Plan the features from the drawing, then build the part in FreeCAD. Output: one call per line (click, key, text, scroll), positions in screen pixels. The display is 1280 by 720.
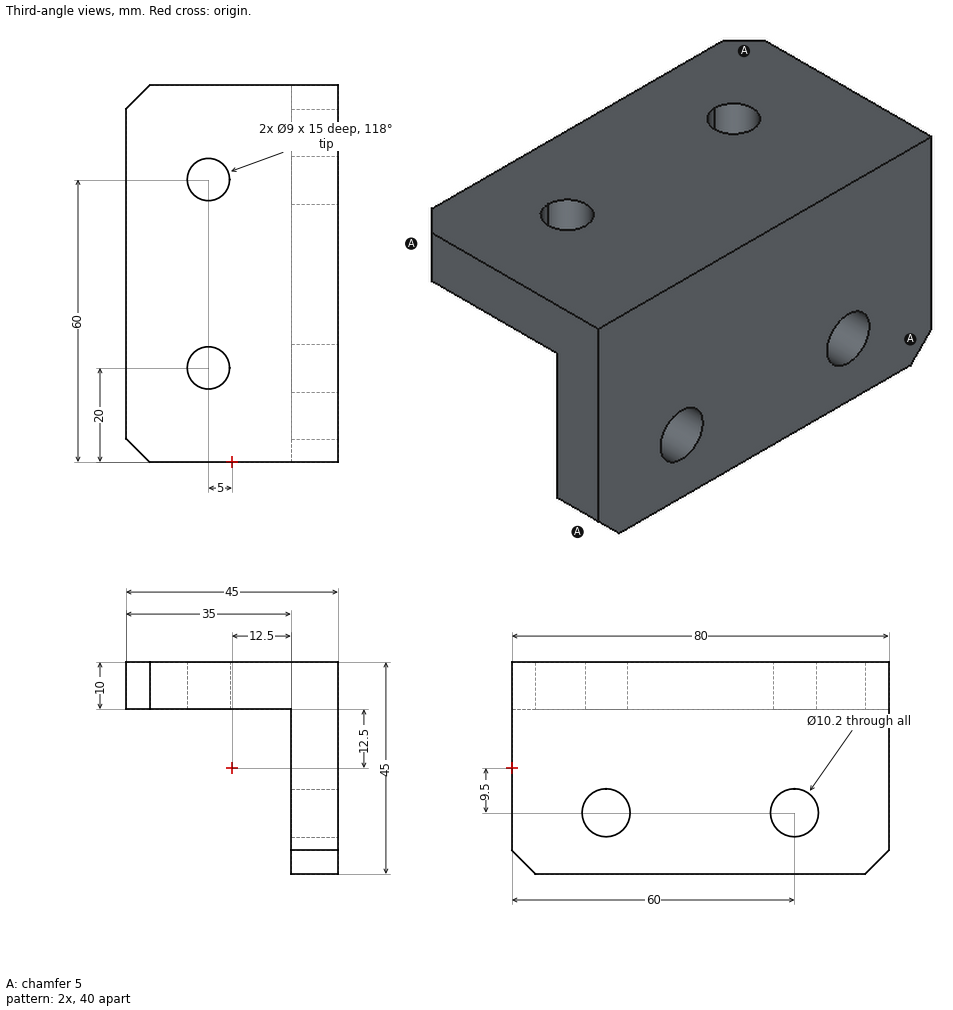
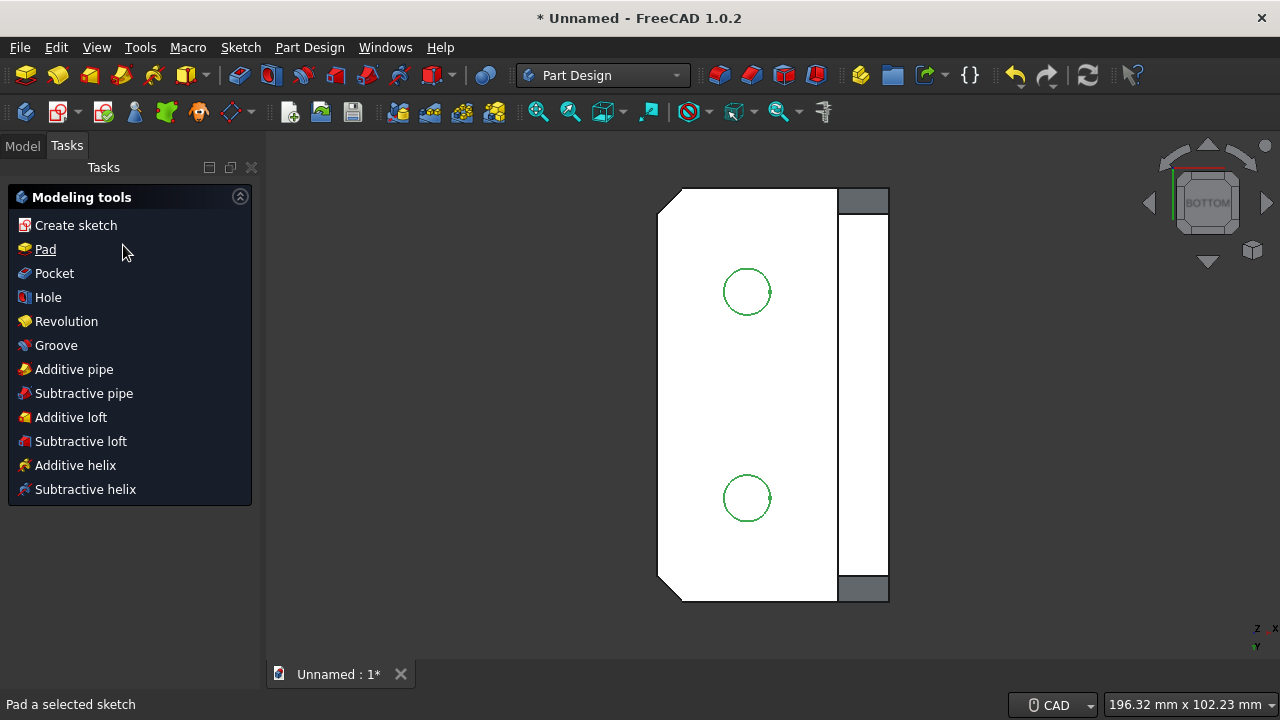
click(272, 76)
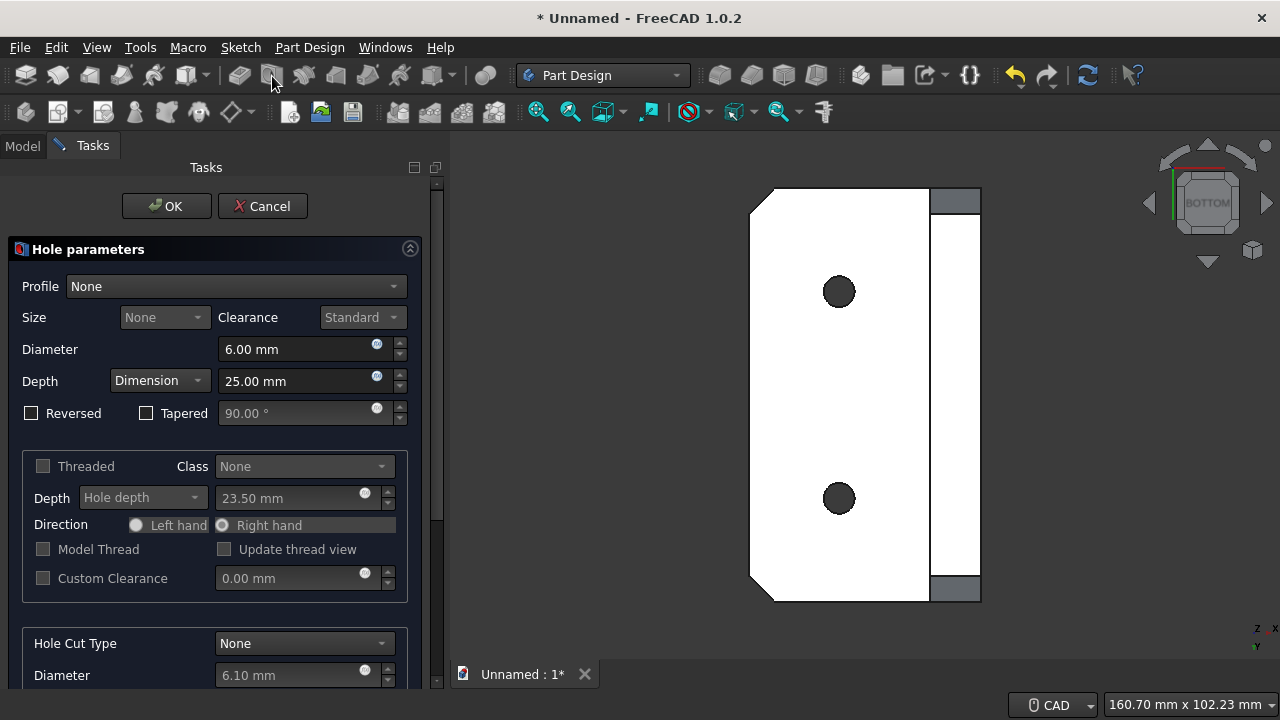
triple_click(305, 349)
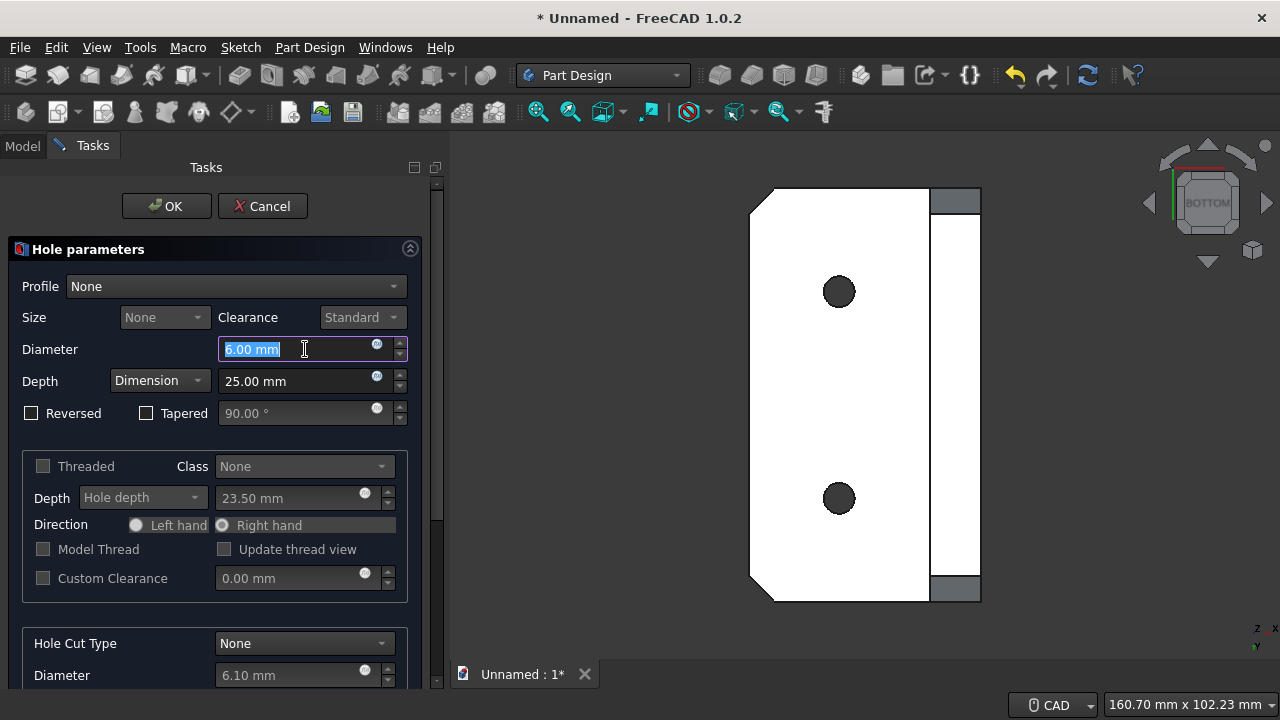
text(9)
key(Tab)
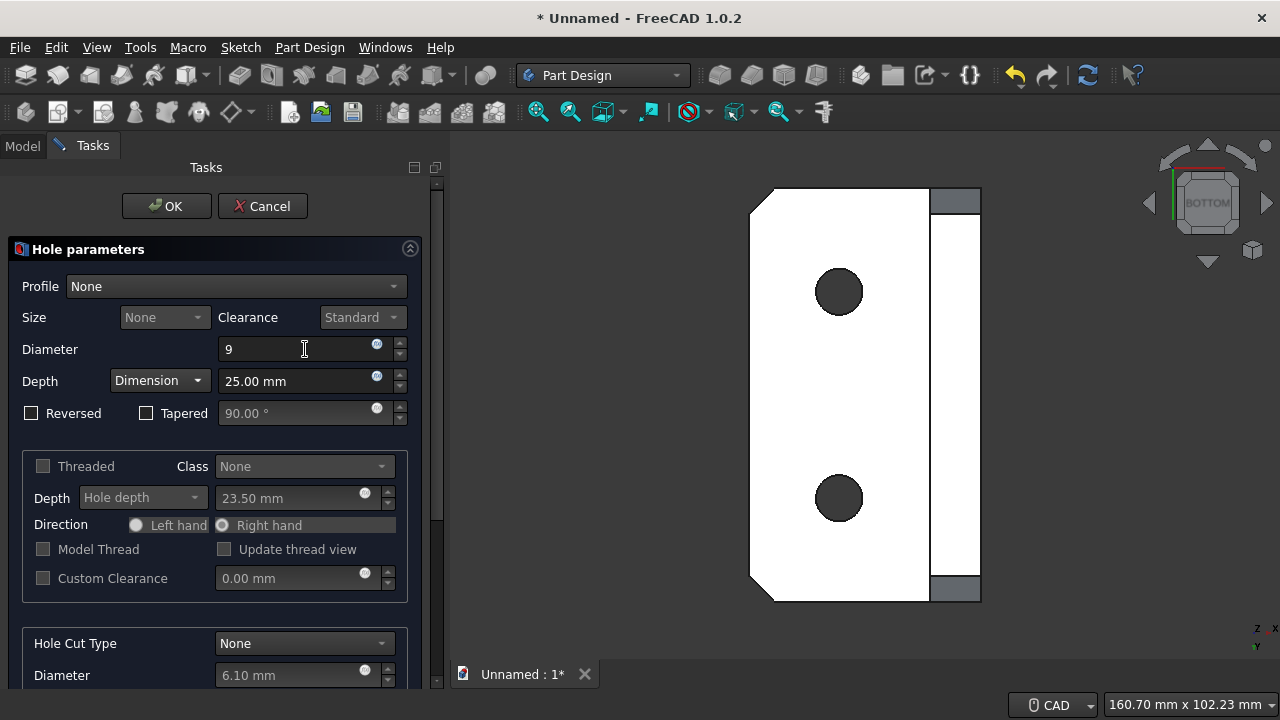
triple_click(305, 381)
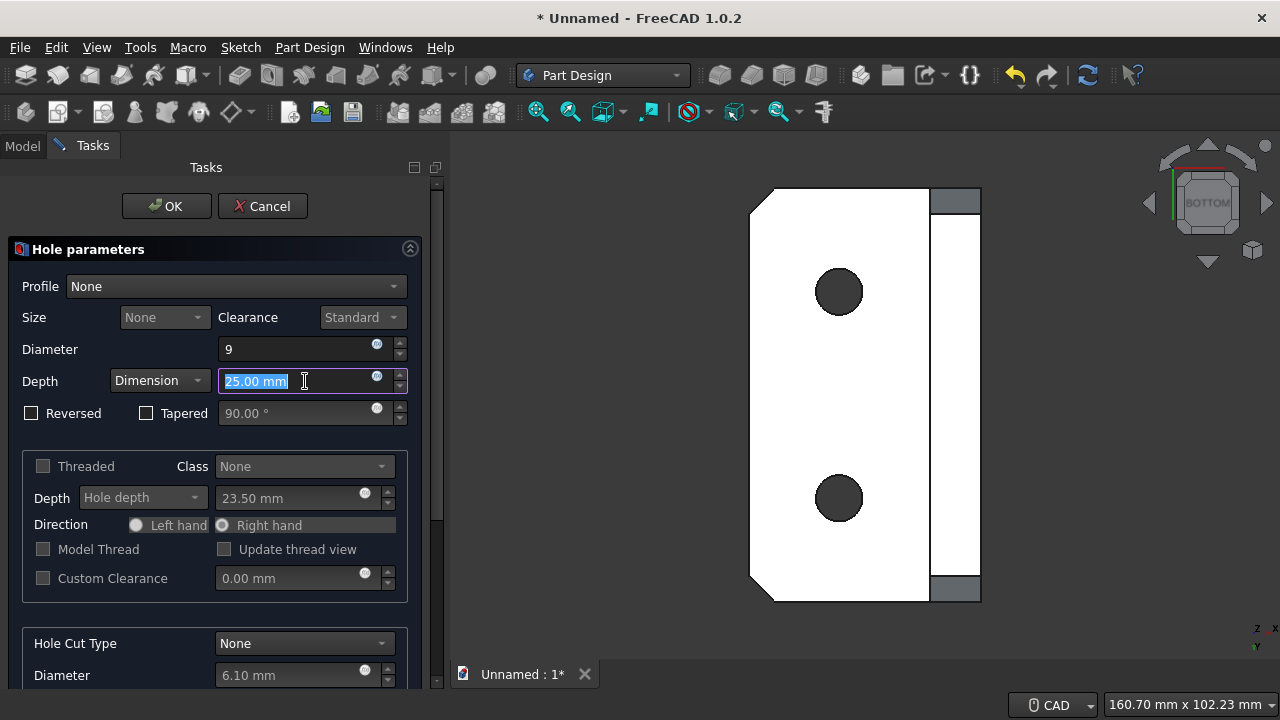
text(15)
key(Tab)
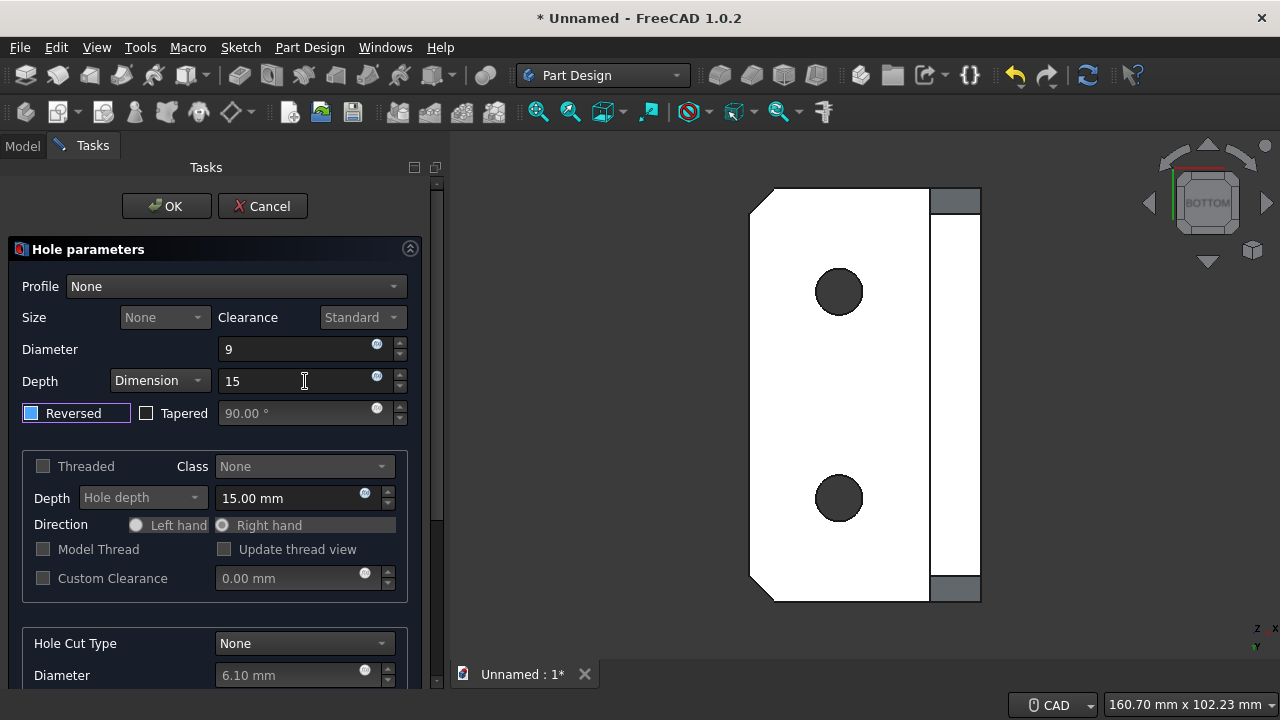
click(167, 206)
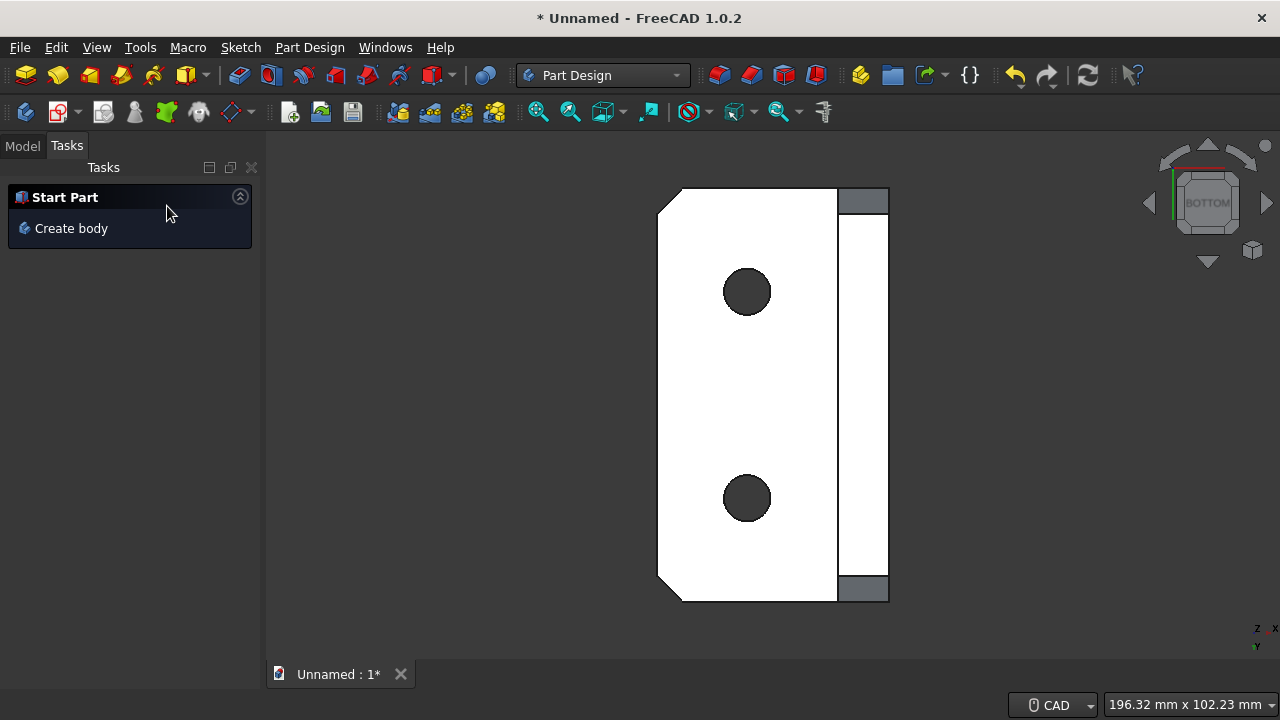
key(6)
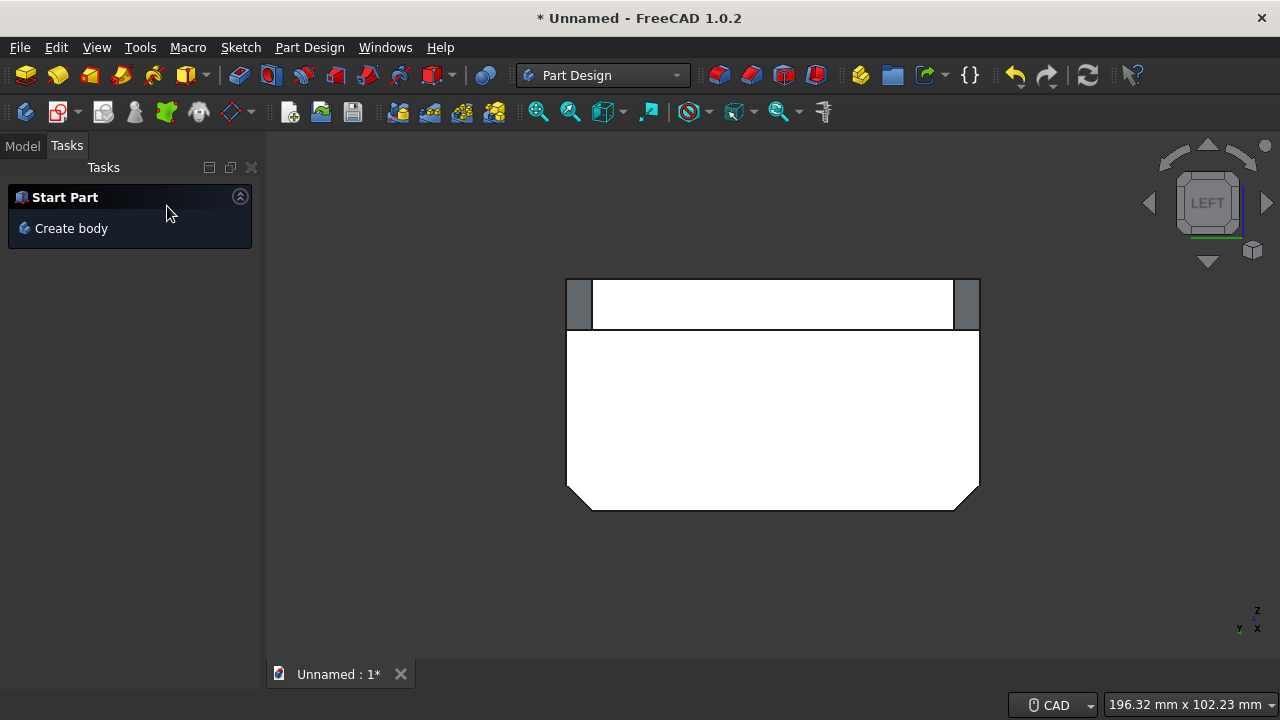
key(v)
key(f)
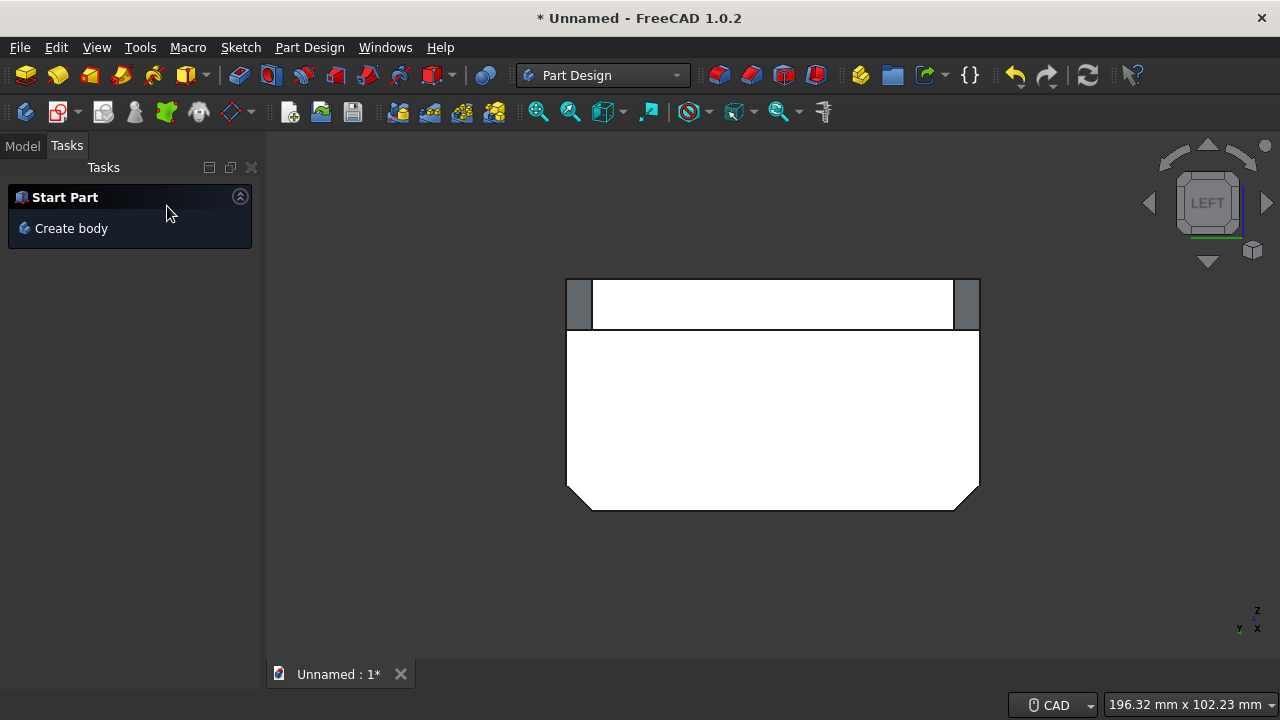
click(714, 420)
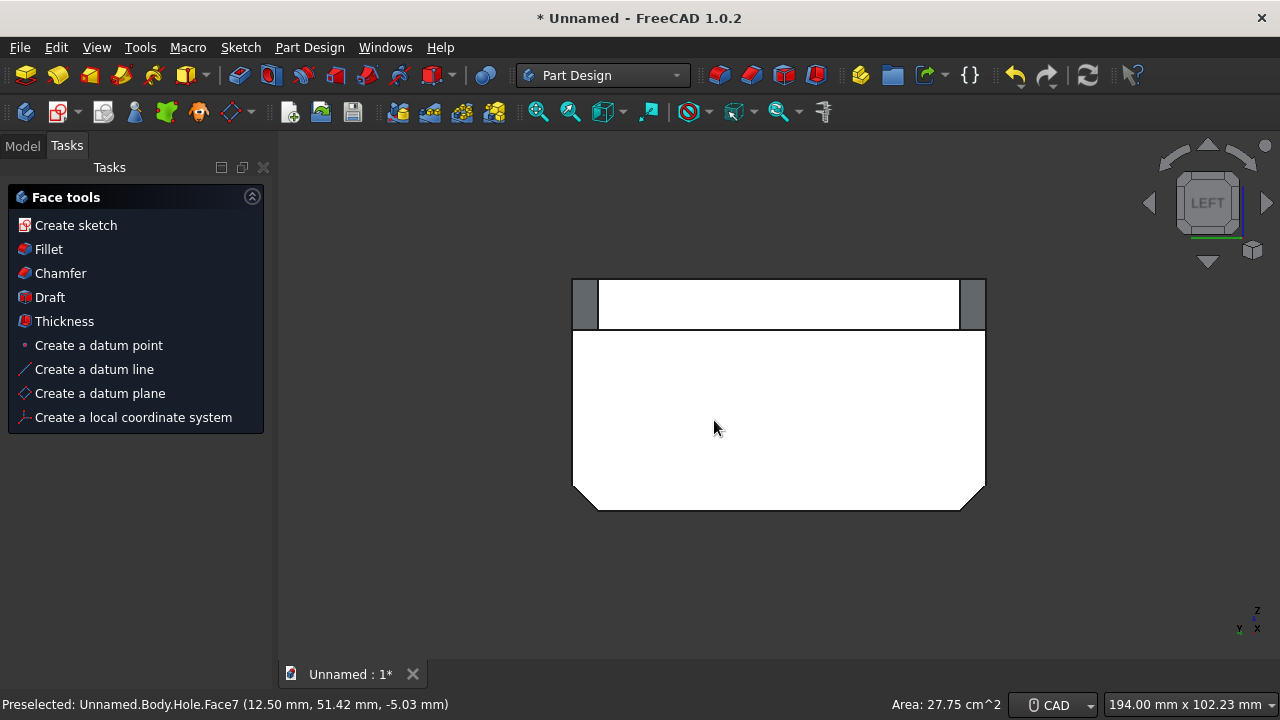
click(58, 112)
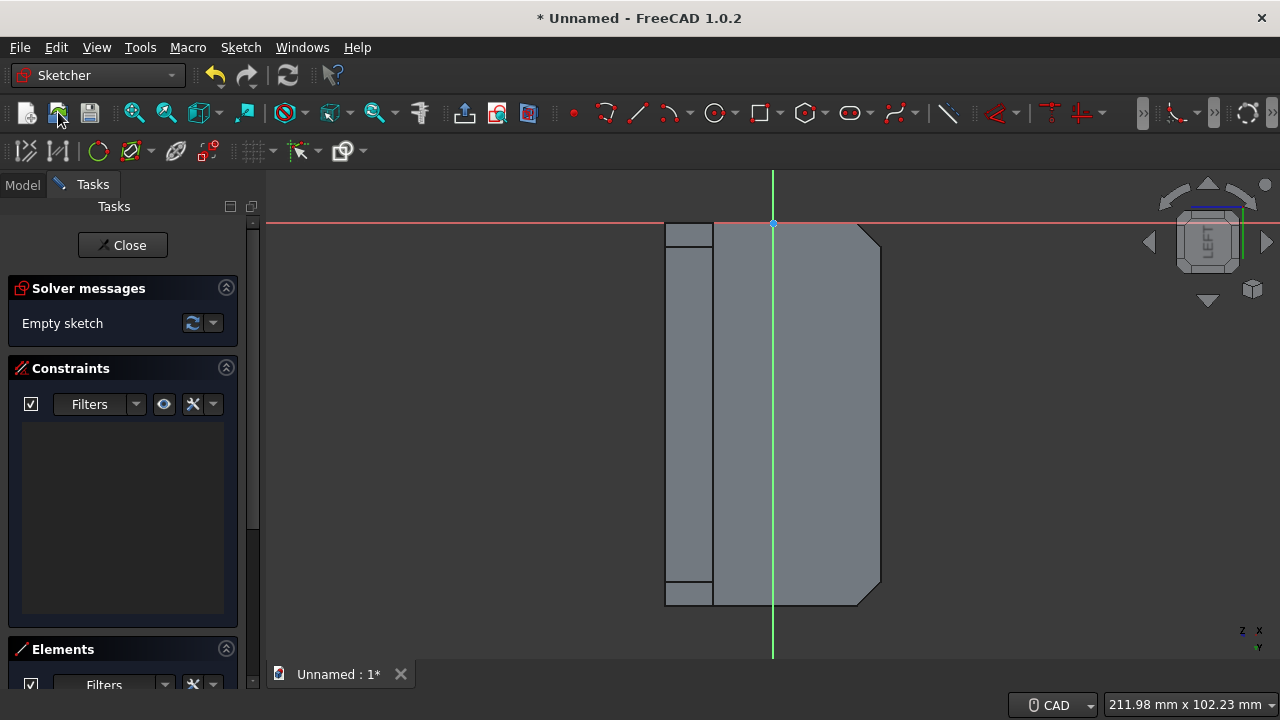
scroll(841, 529, up, 9)